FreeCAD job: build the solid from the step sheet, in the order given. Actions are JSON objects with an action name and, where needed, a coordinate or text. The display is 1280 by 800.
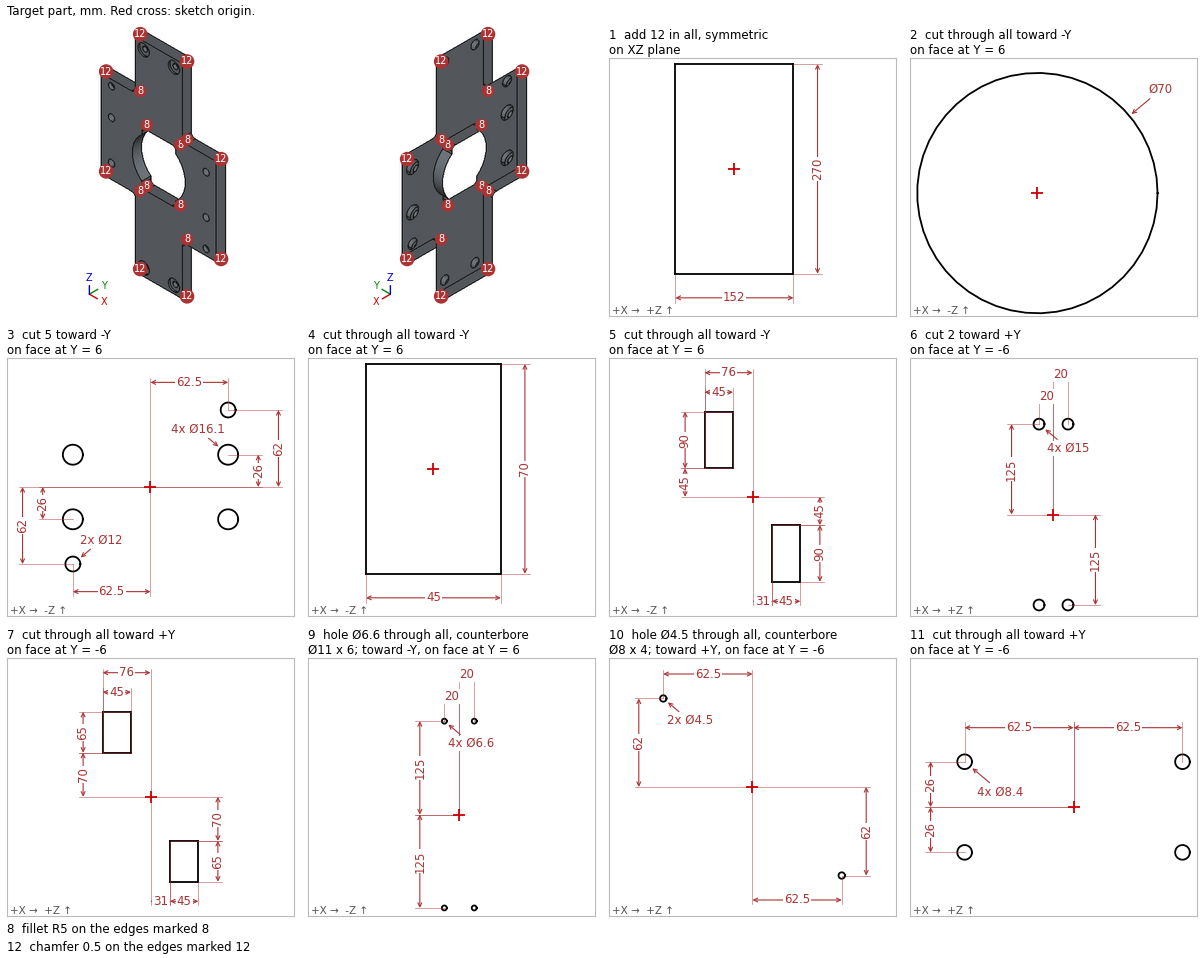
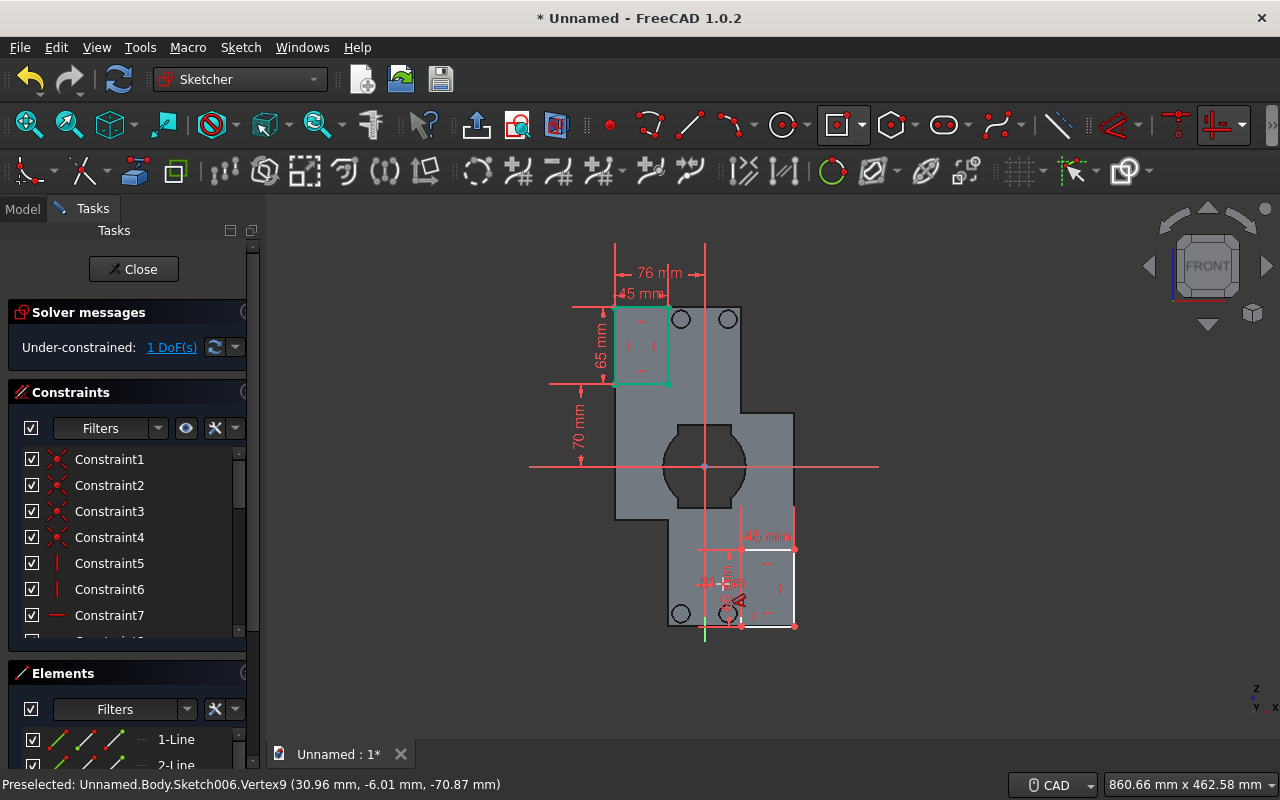
{"action": "left_click", "coordinate": [741, 550]}
{"action": "left_click", "coordinate": [775, 508]}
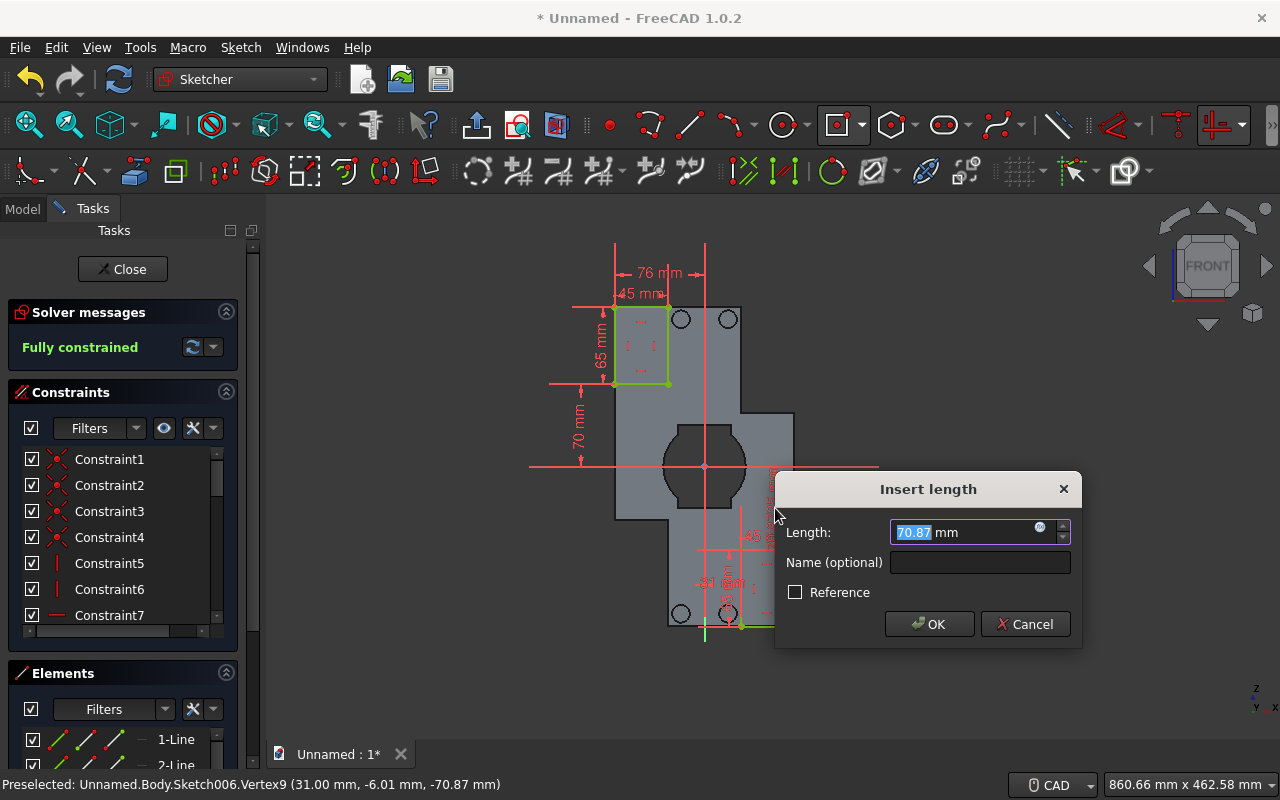
{"action": "type", "text": "70"}
{"action": "key", "text": "Return"}
{"action": "key", "text": "Escape"}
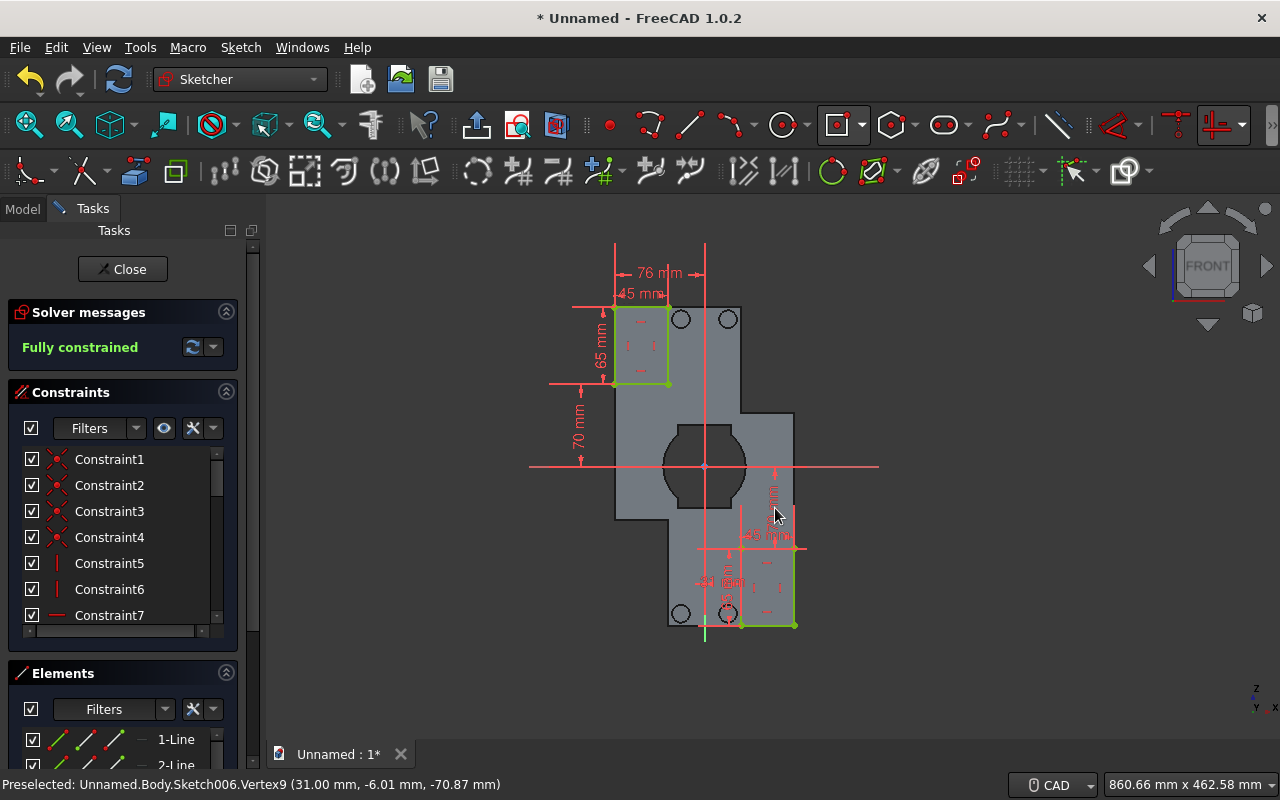
{"action": "left_click", "coordinate": [123, 269]}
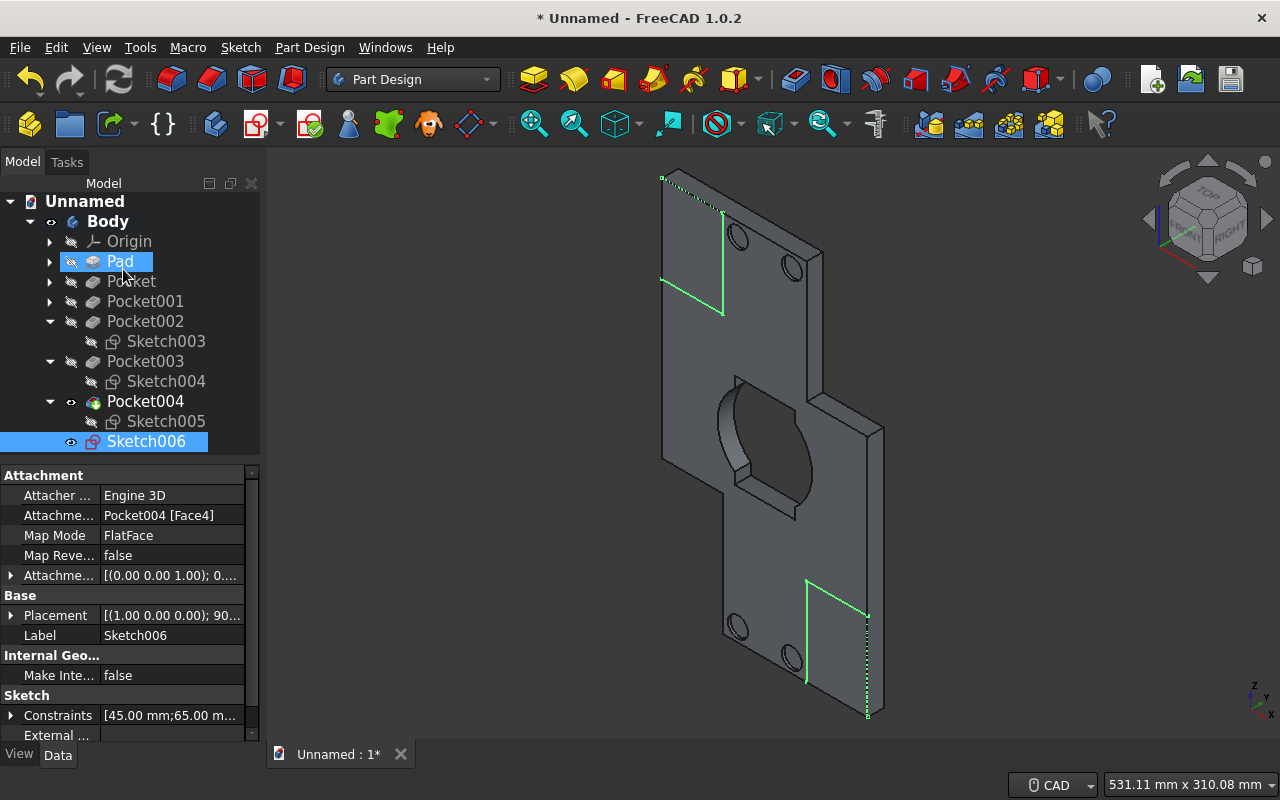
{"action": "left_click", "coordinate": [796, 80]}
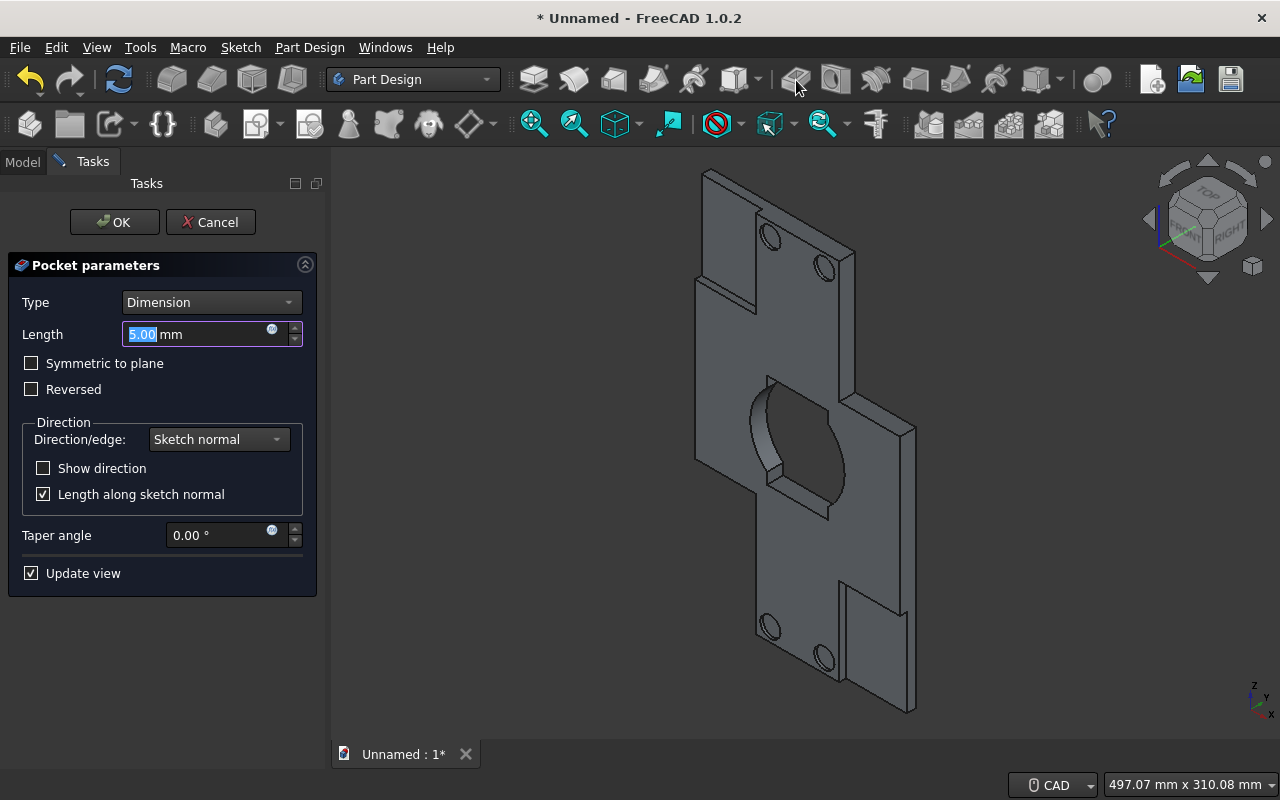
{"action": "left_click", "coordinate": [212, 302]}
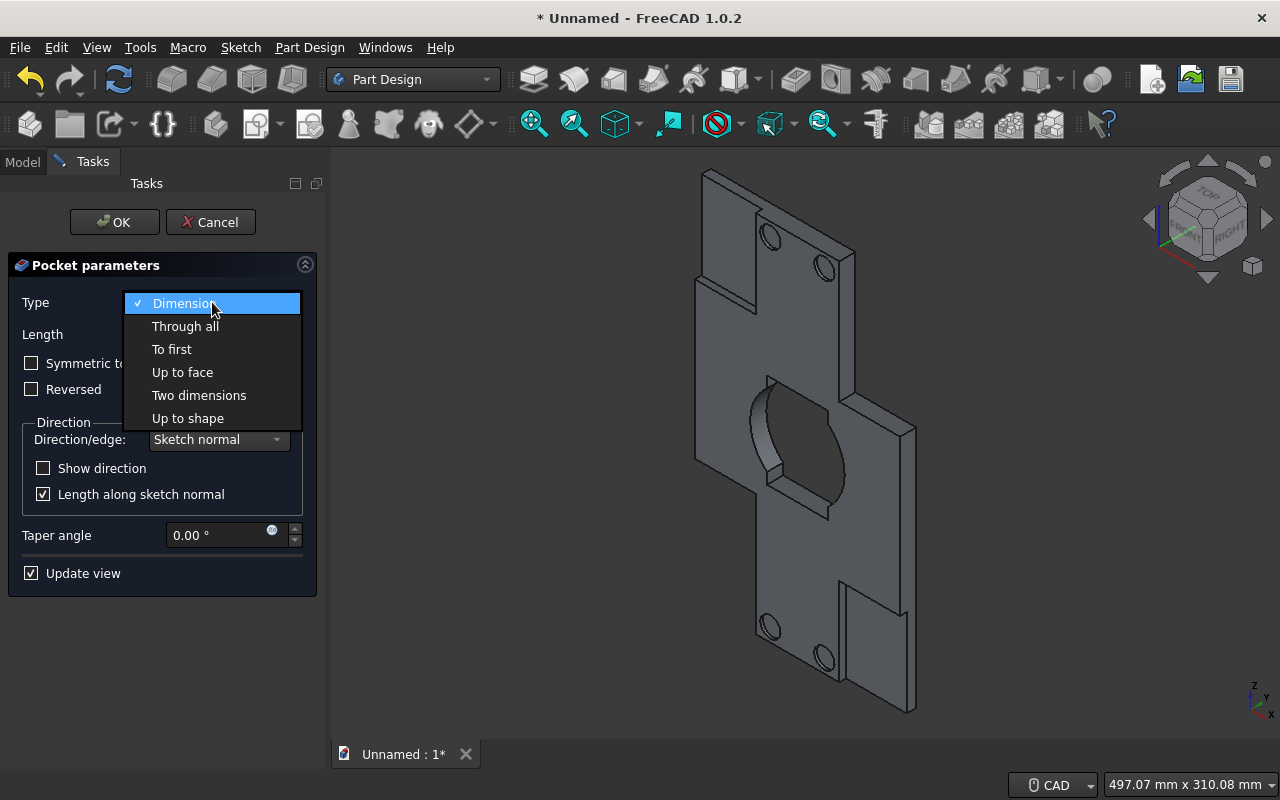
{"action": "left_click", "coordinate": [212, 326]}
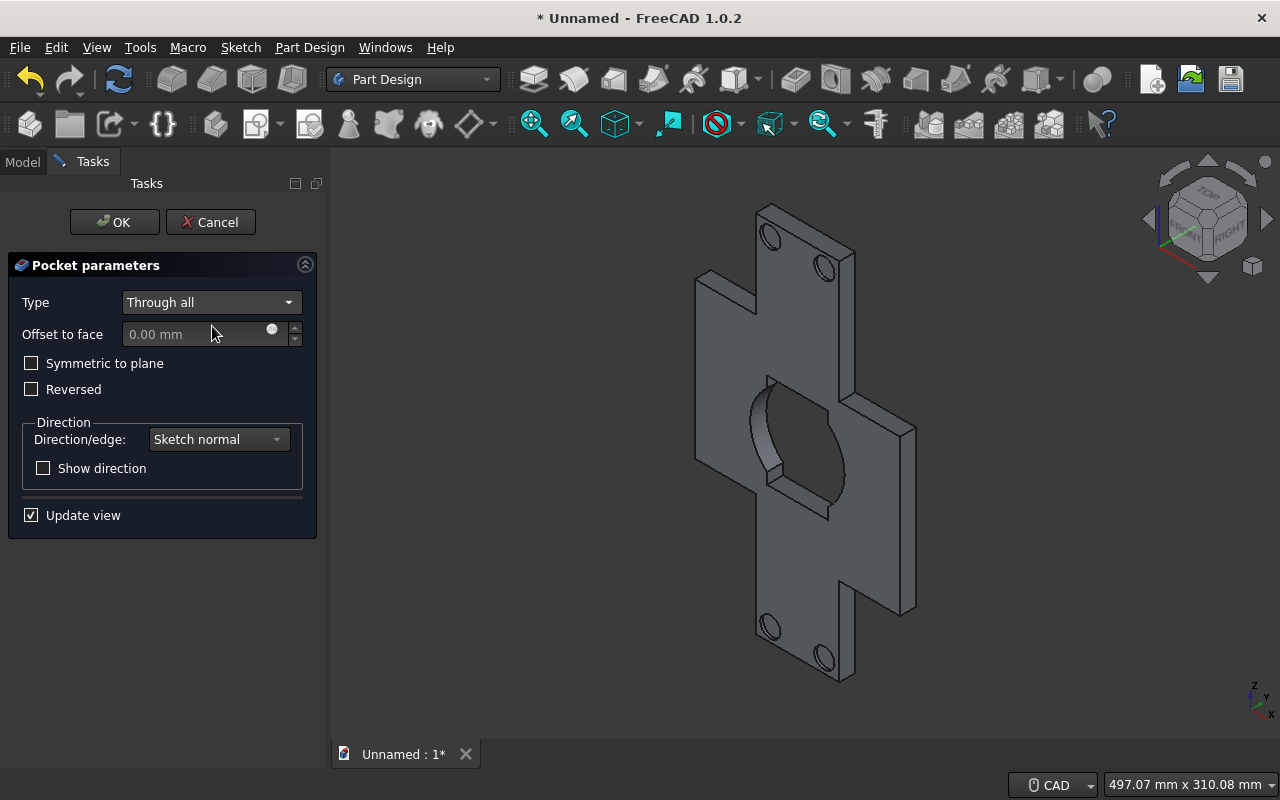
{"action": "left_click", "coordinate": [115, 222]}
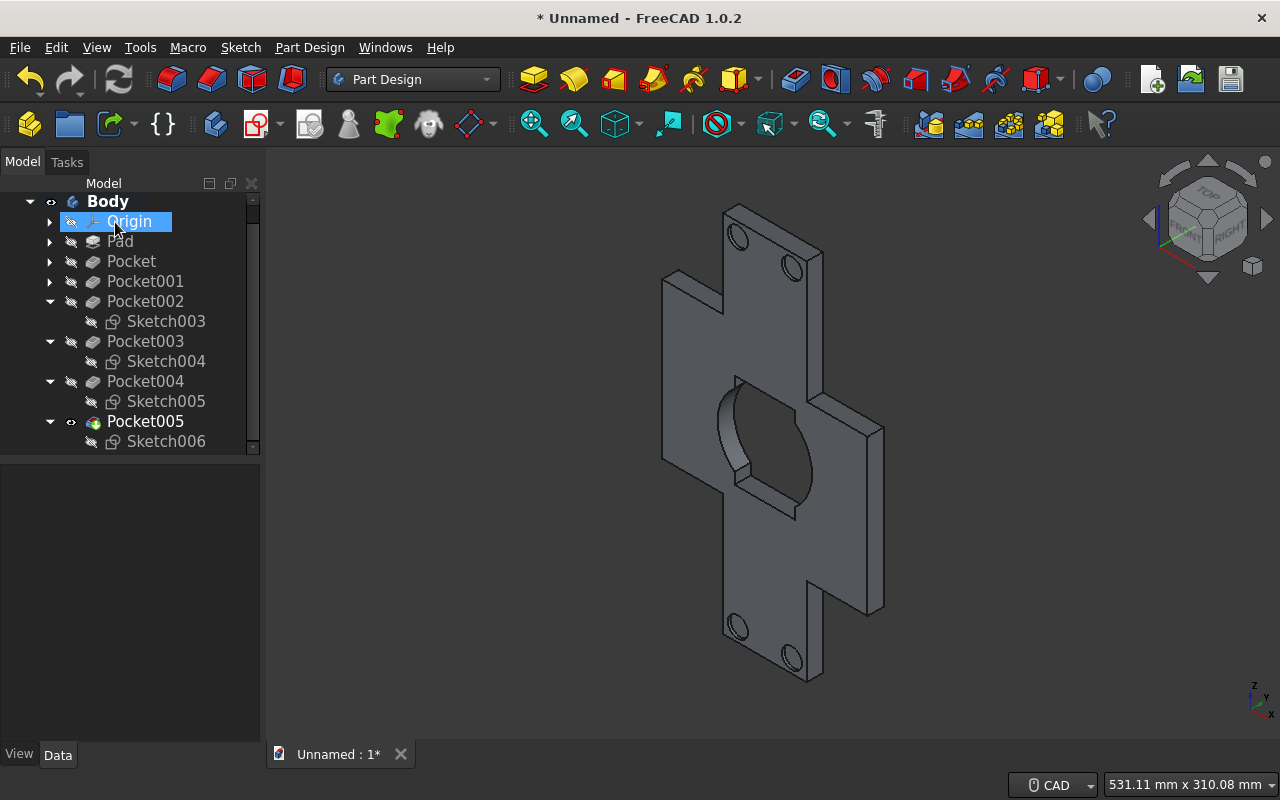
{"action": "key", "text": "2"}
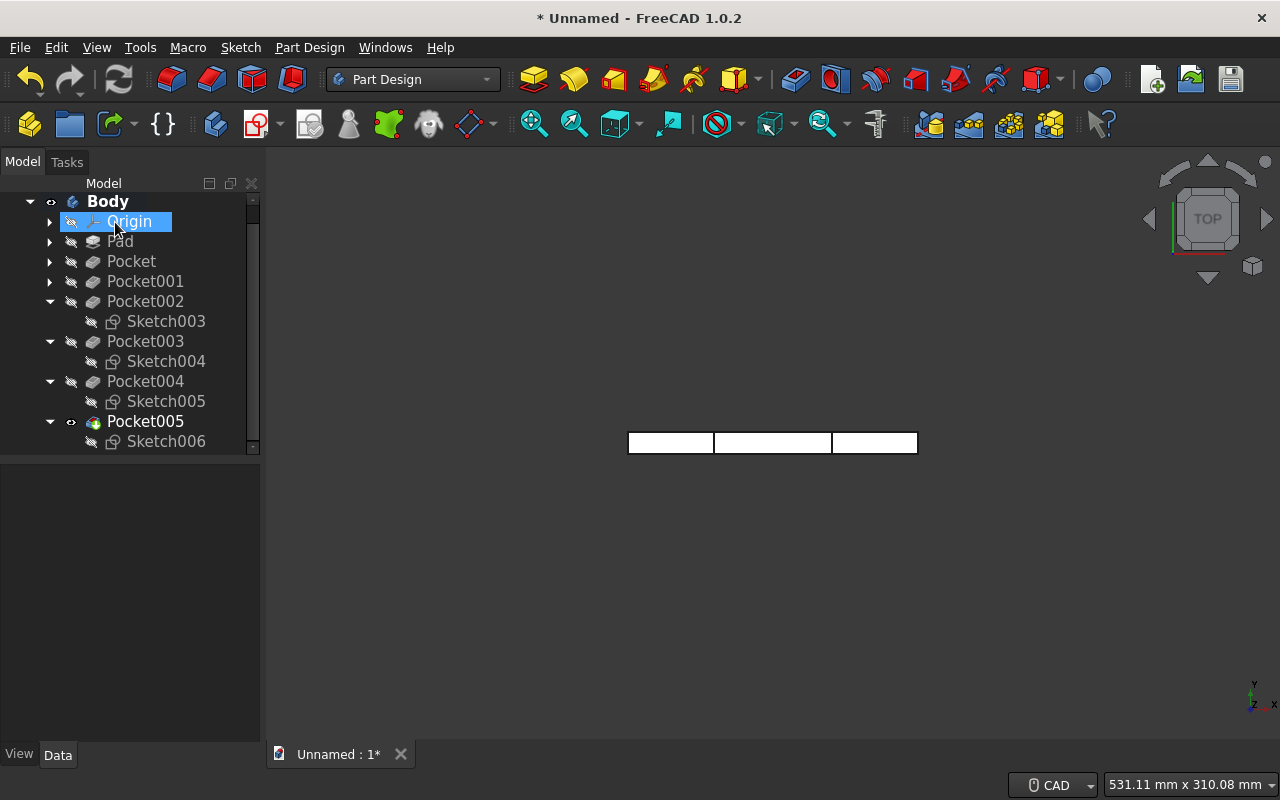
{"action": "key", "text": "v f"}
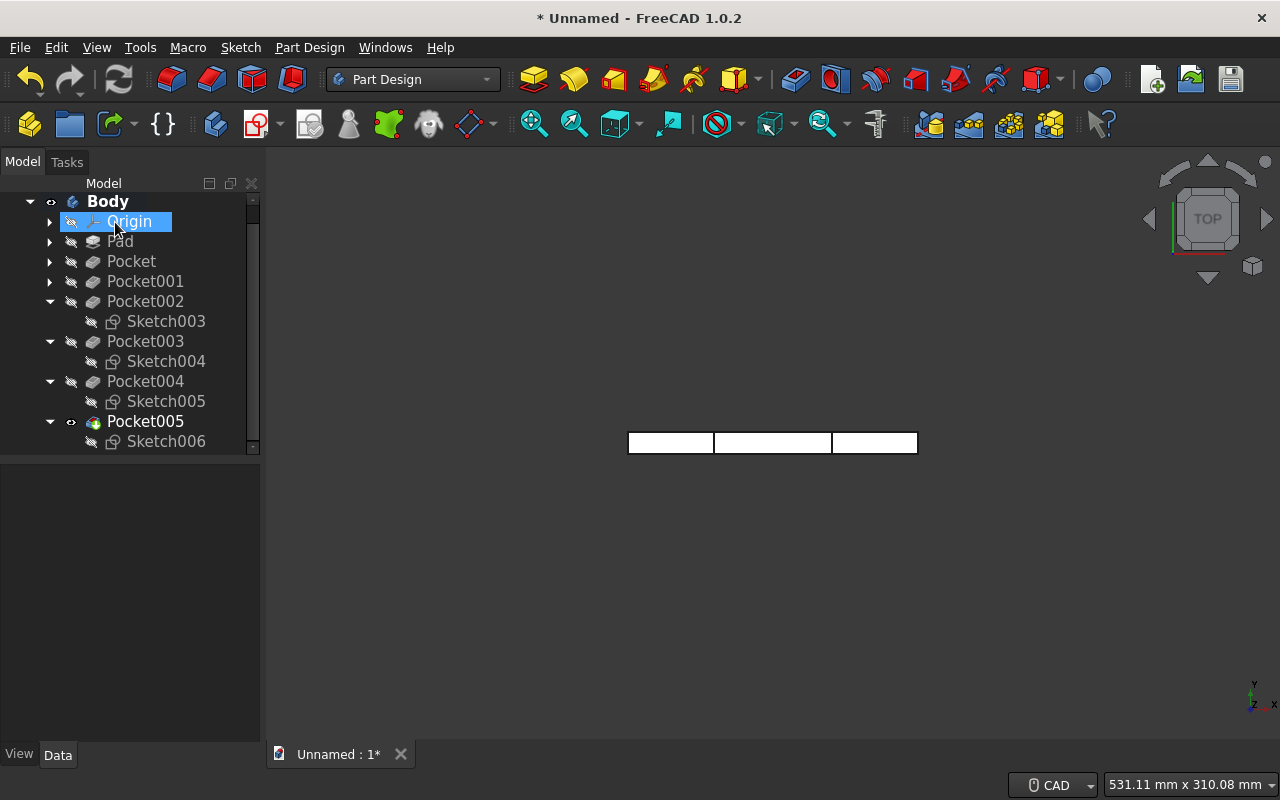
{"action": "key", "text": "0"}